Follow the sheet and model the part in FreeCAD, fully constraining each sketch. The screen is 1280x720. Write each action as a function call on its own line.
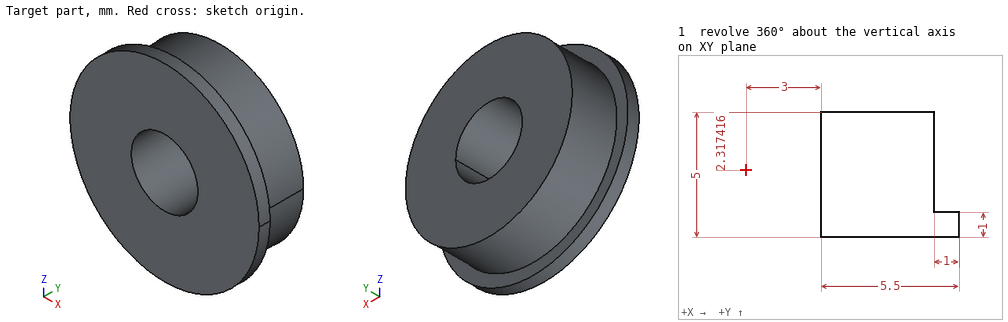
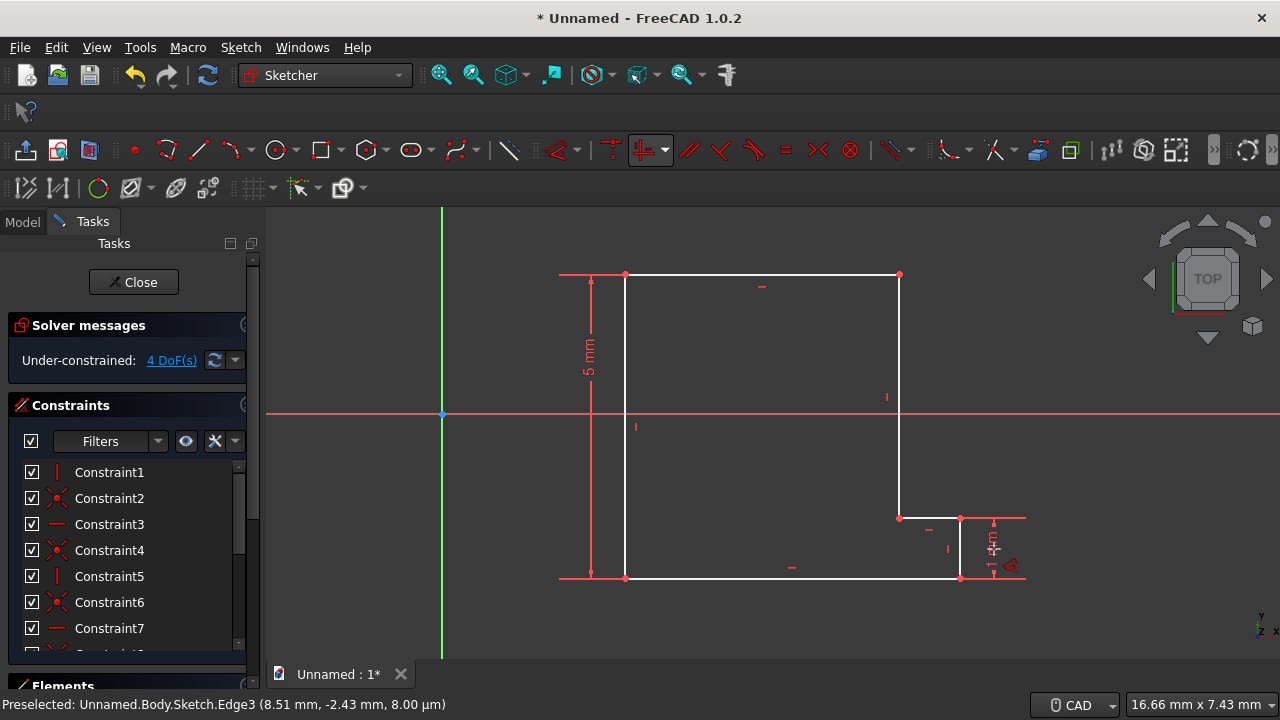
click(942, 518)
click(915, 552)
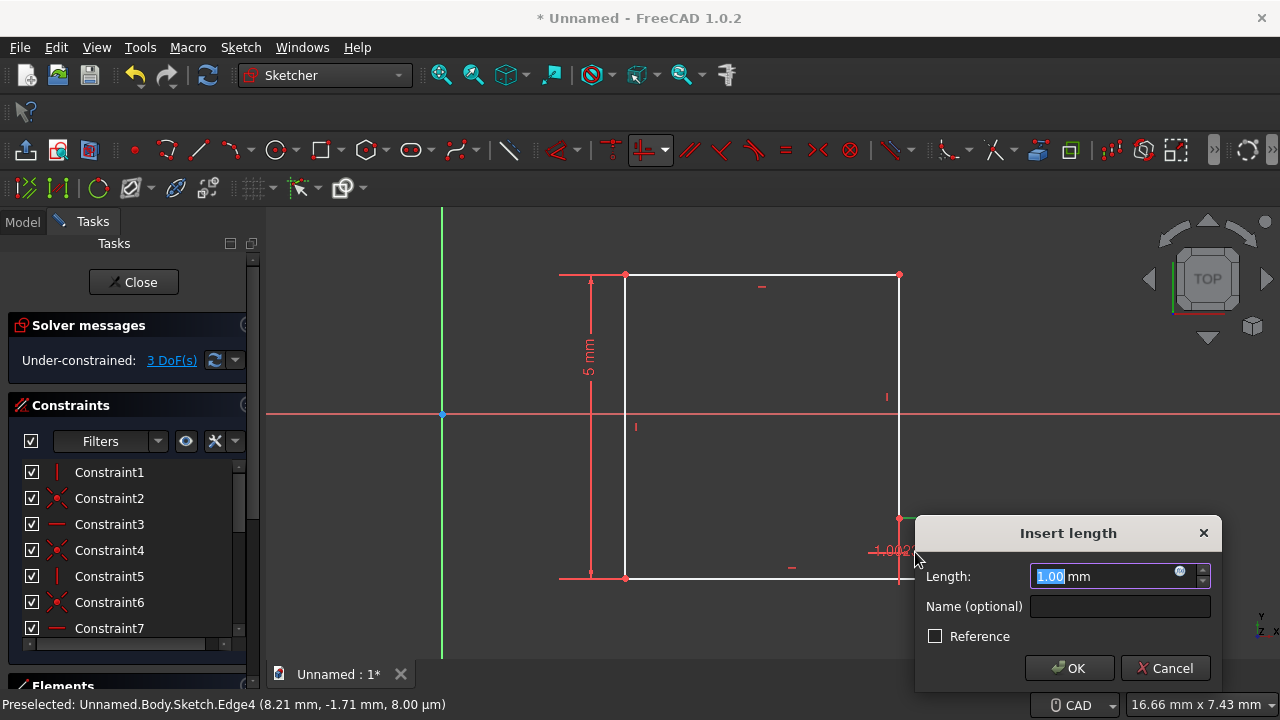
text(1)
key(Return)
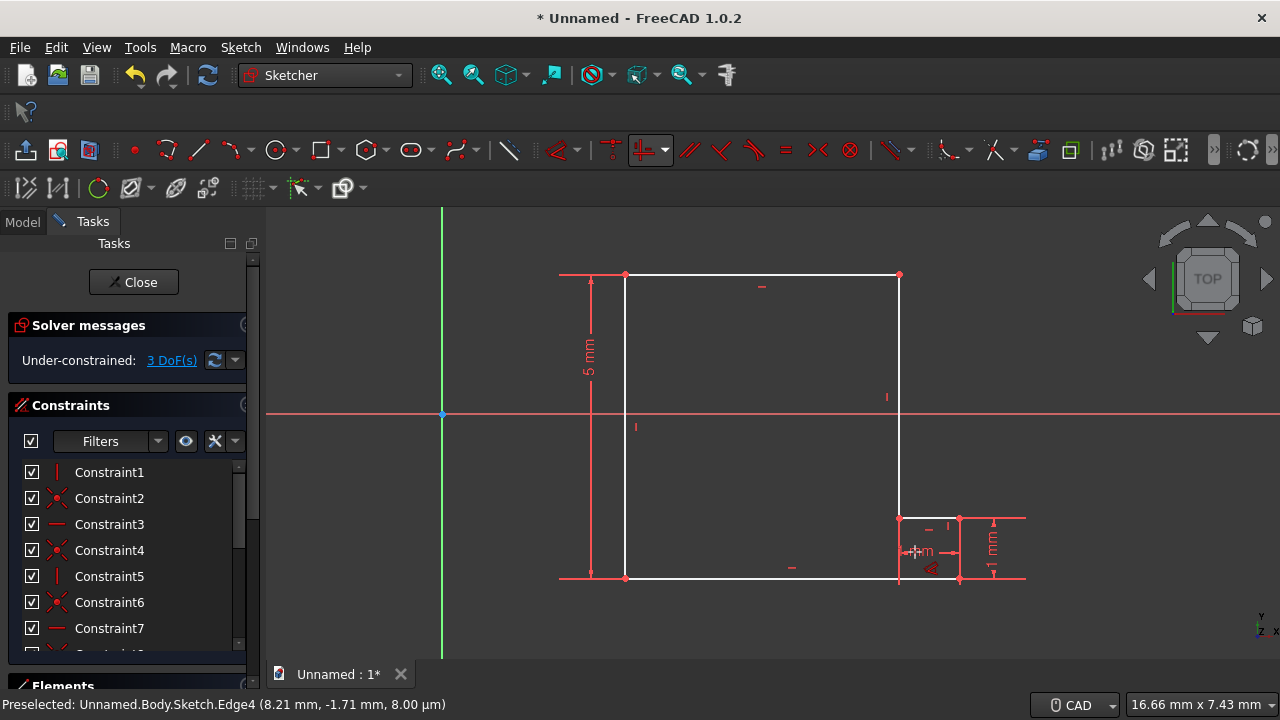
click(625, 275)
click(534, 241)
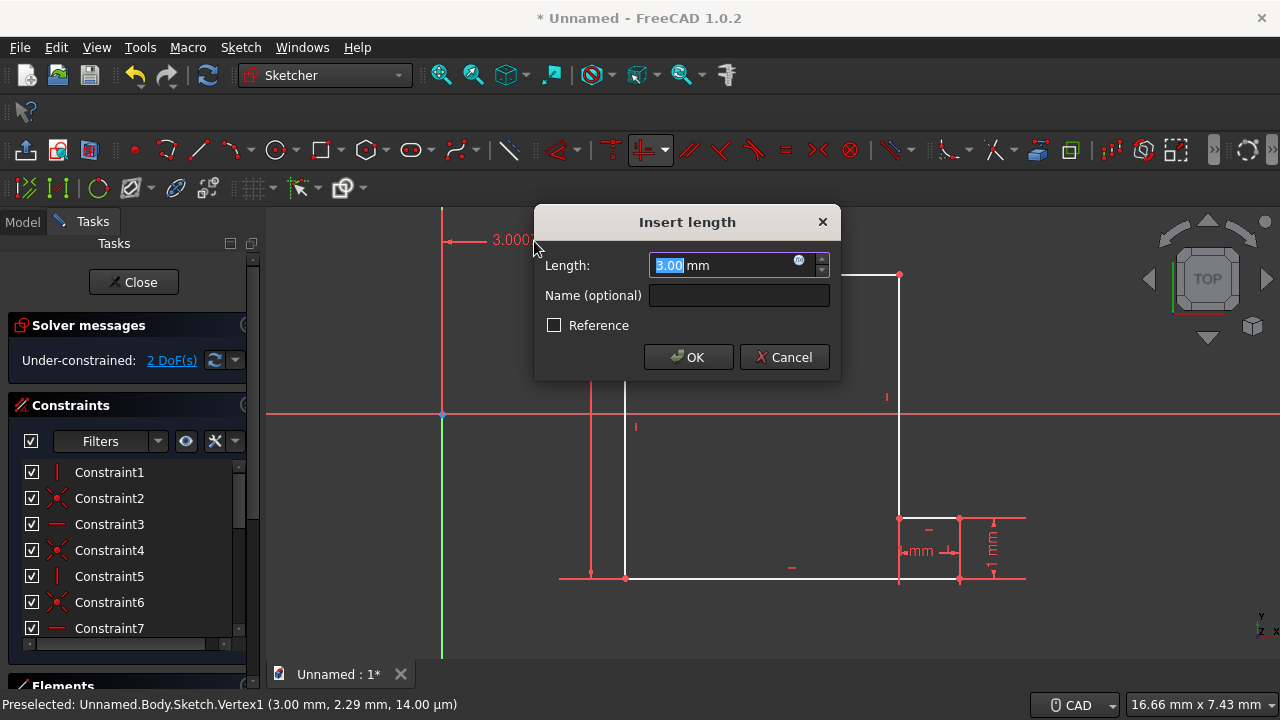
text(3)
key(Return)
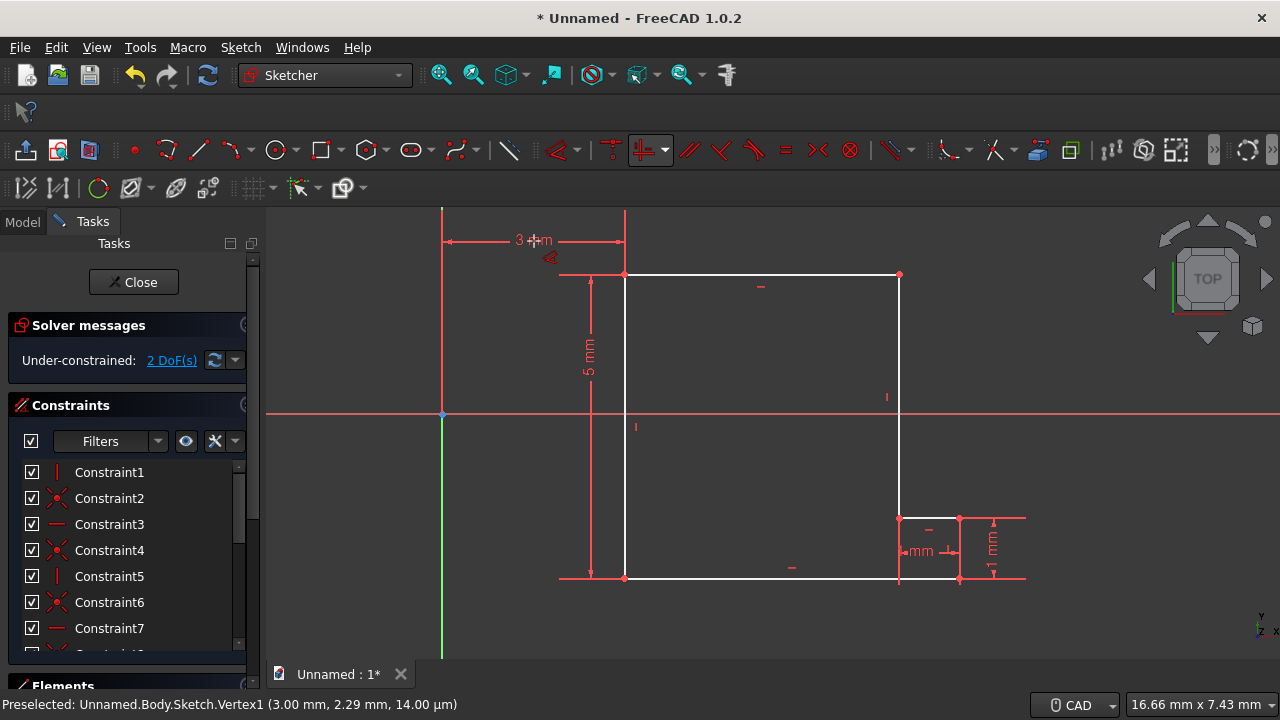
click(725, 579)
click(792, 613)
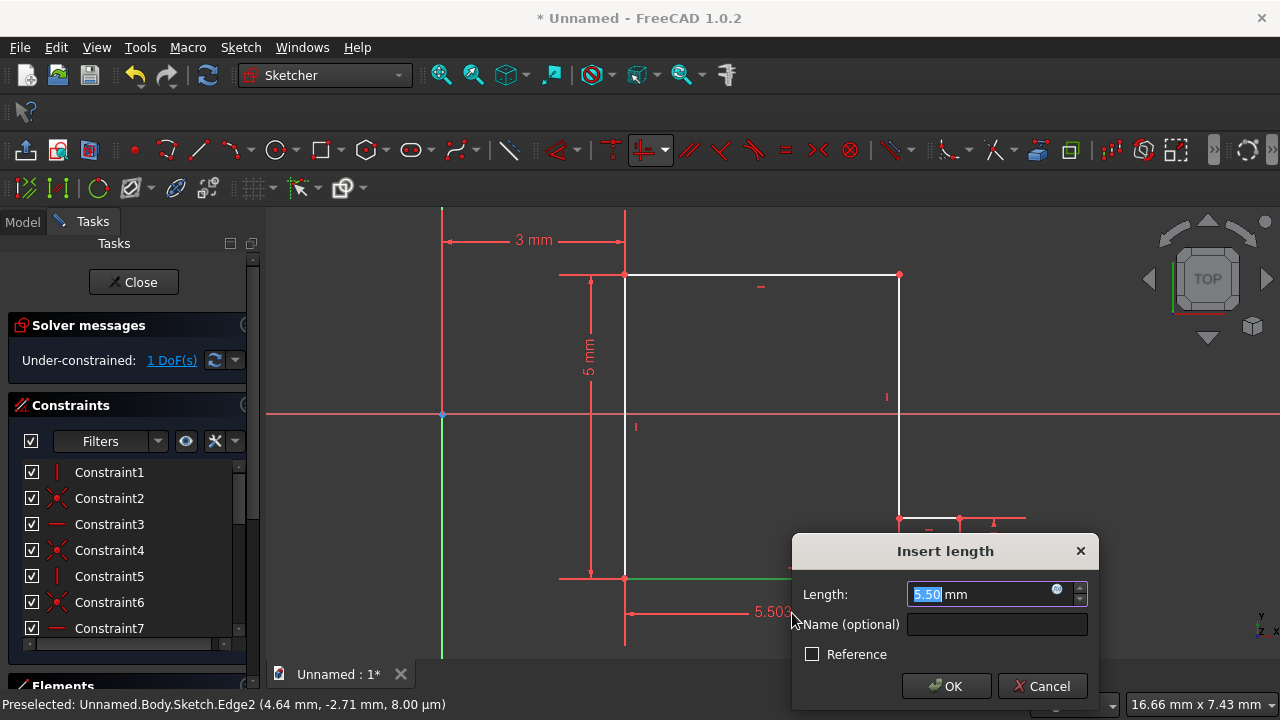
text(5.5)
key(Return)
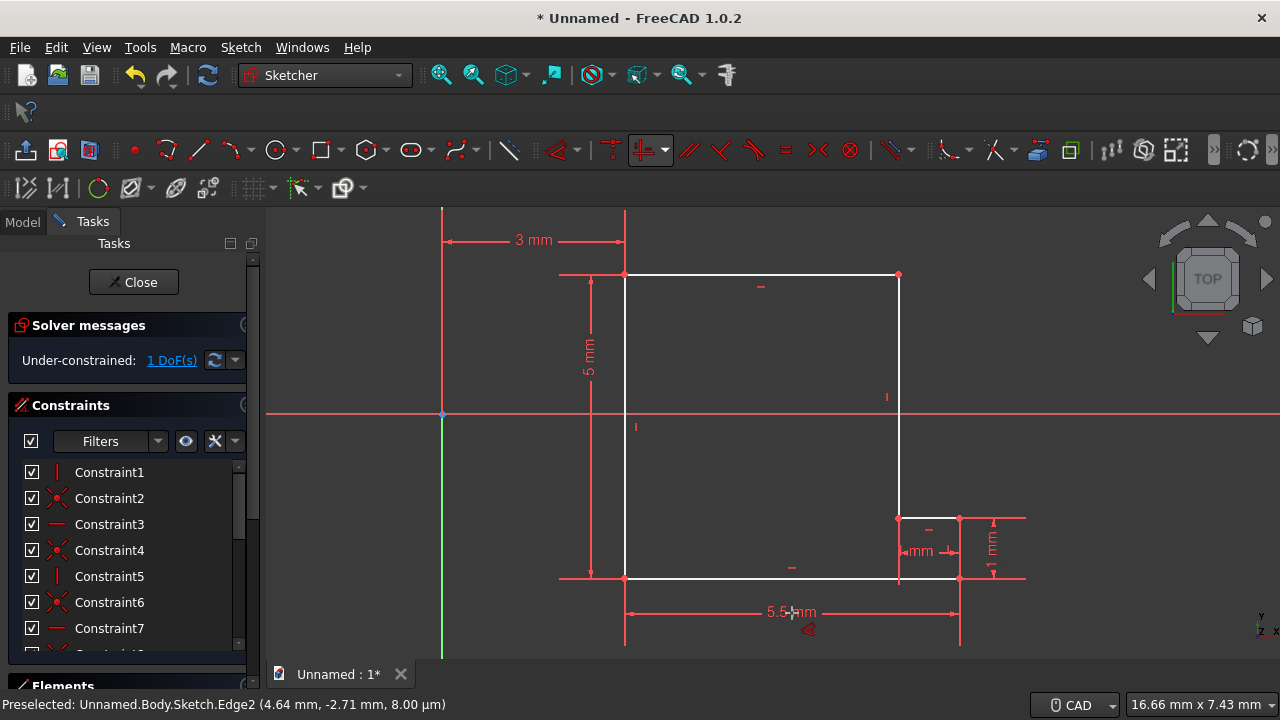
click(625, 275)
click(408, 344)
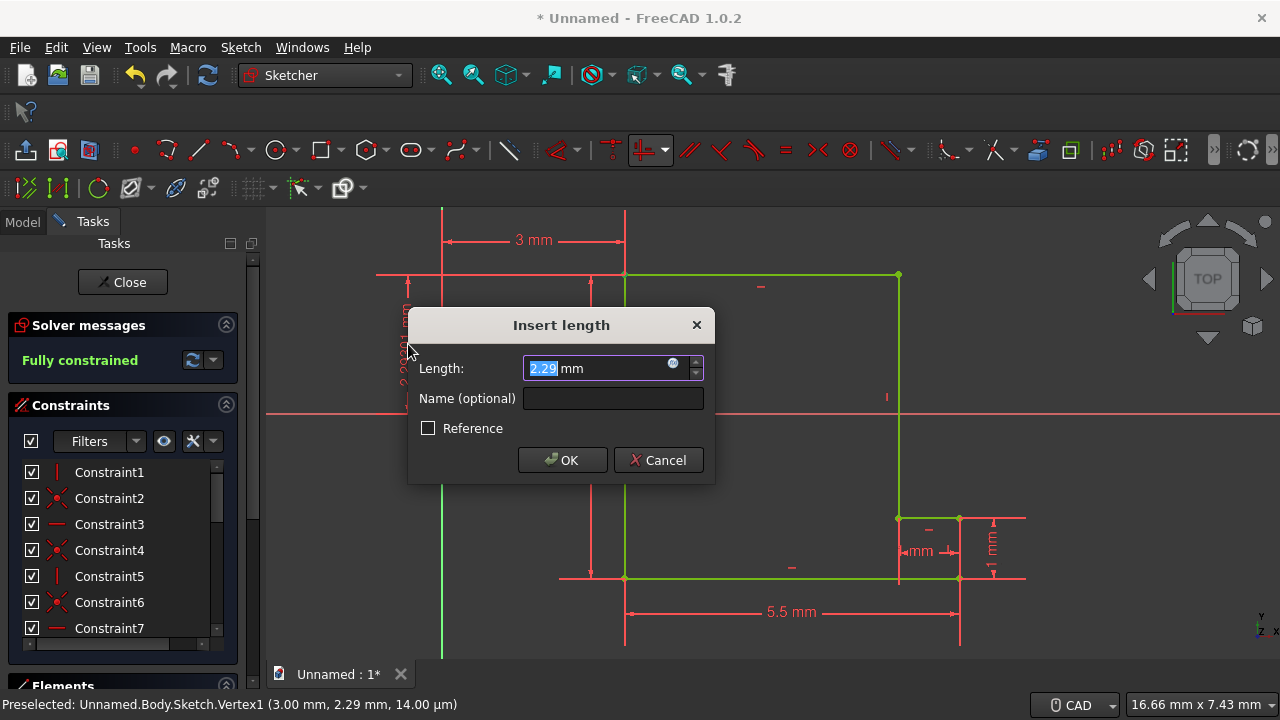
text(2.317416)
key(Return)
key(Escape)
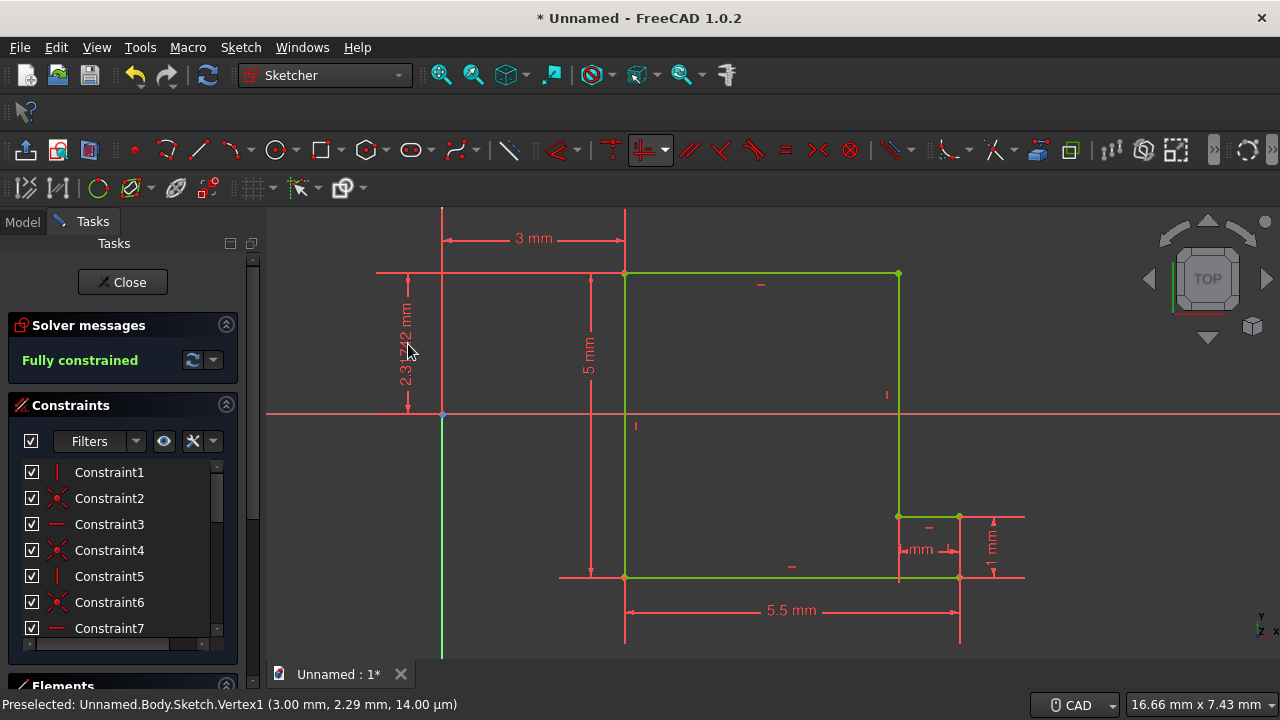
click(123, 282)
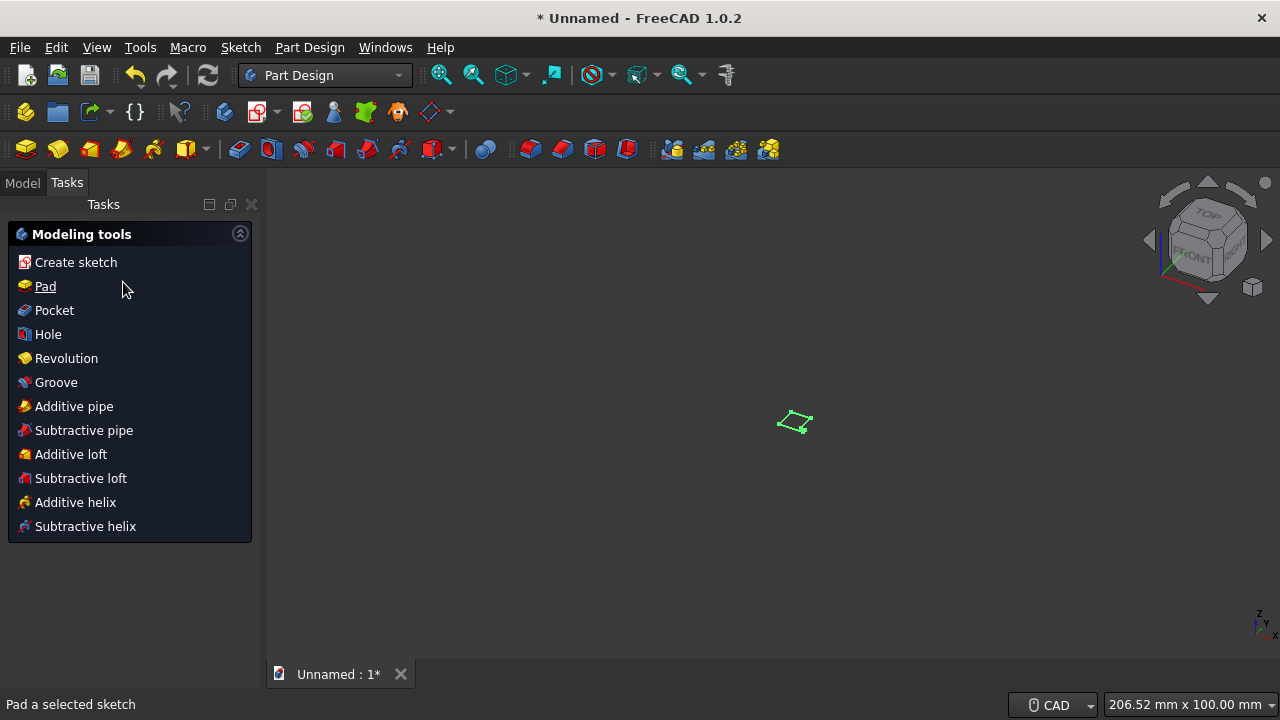
click(58, 150)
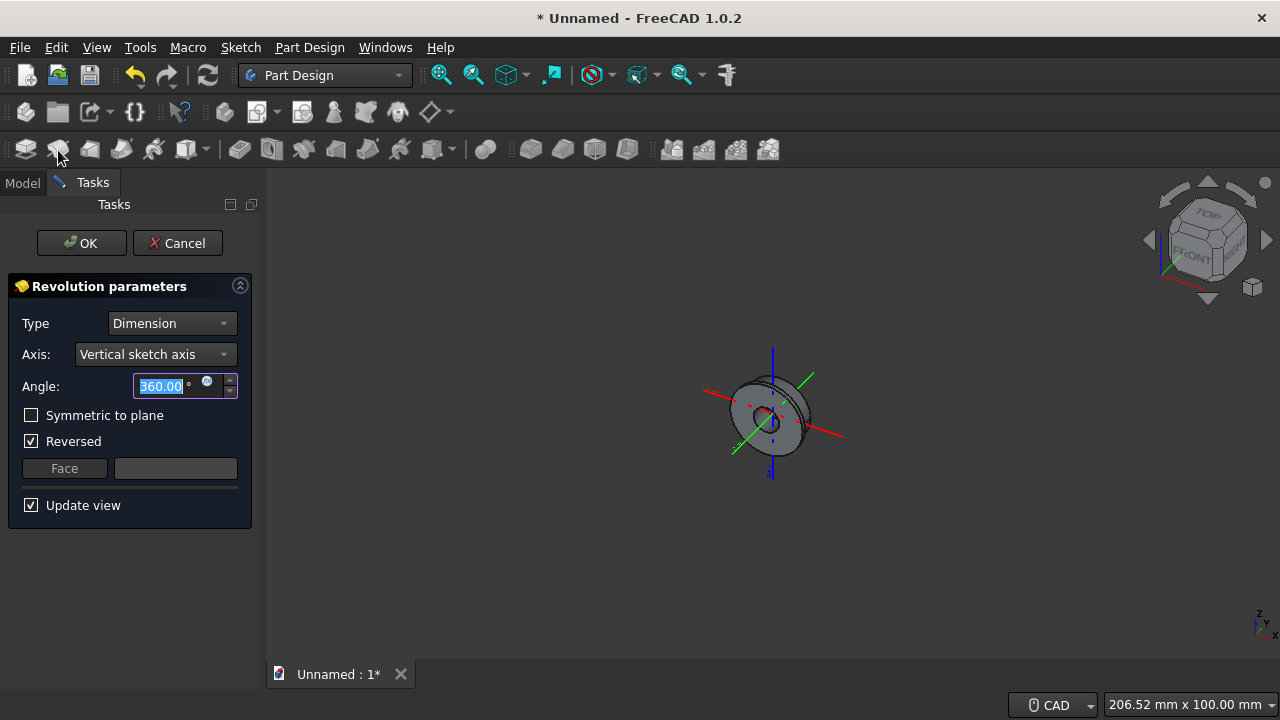
click(82, 243)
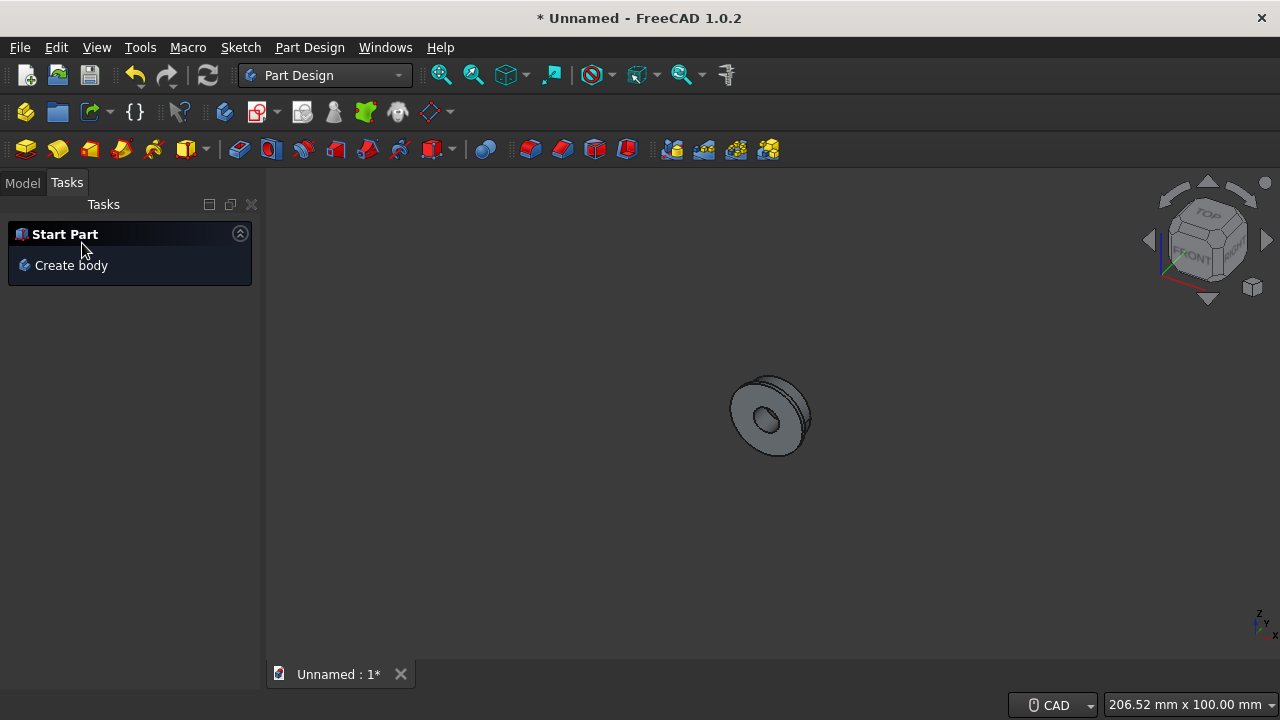
key(0)